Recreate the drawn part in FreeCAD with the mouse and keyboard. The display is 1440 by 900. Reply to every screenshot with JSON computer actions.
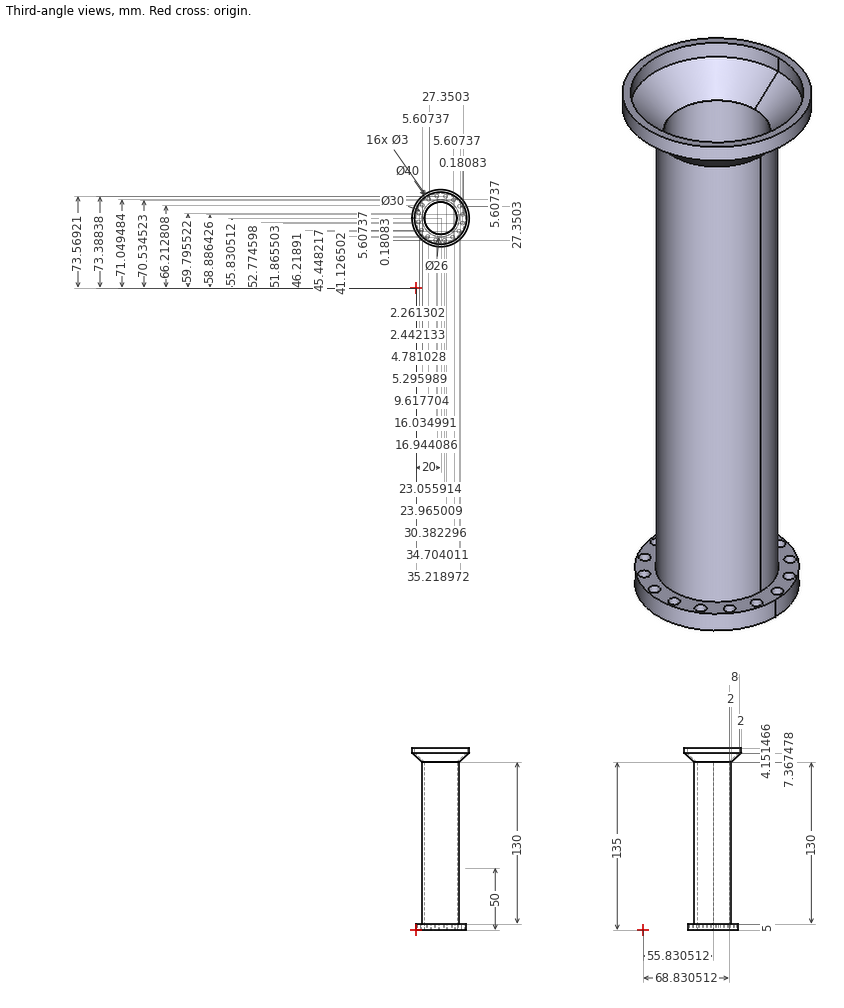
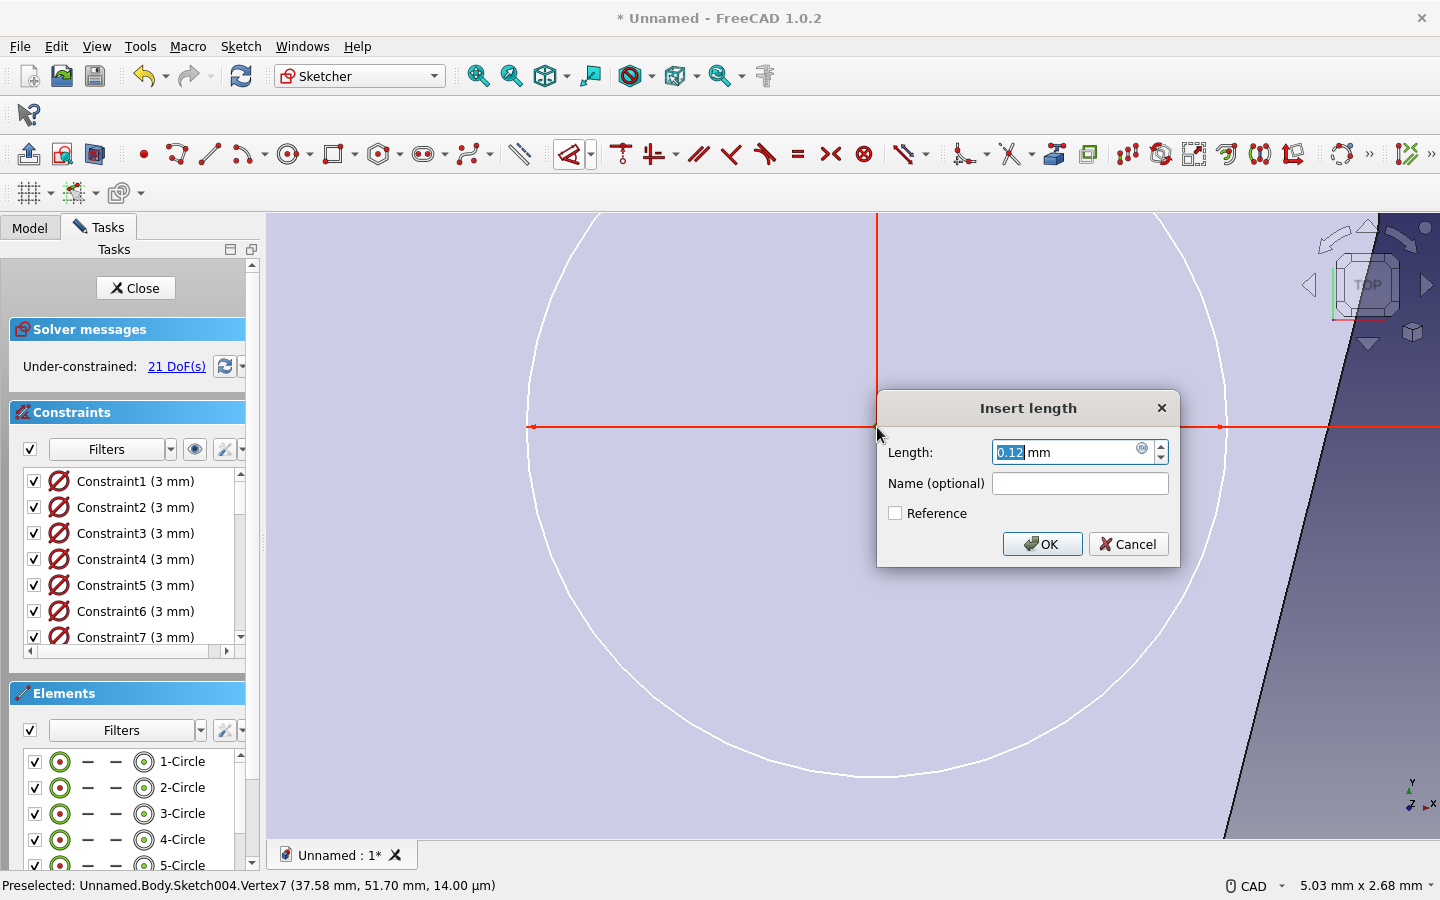
{"action": "type", "text": "0.18083"}
{"action": "key", "text": "Return"}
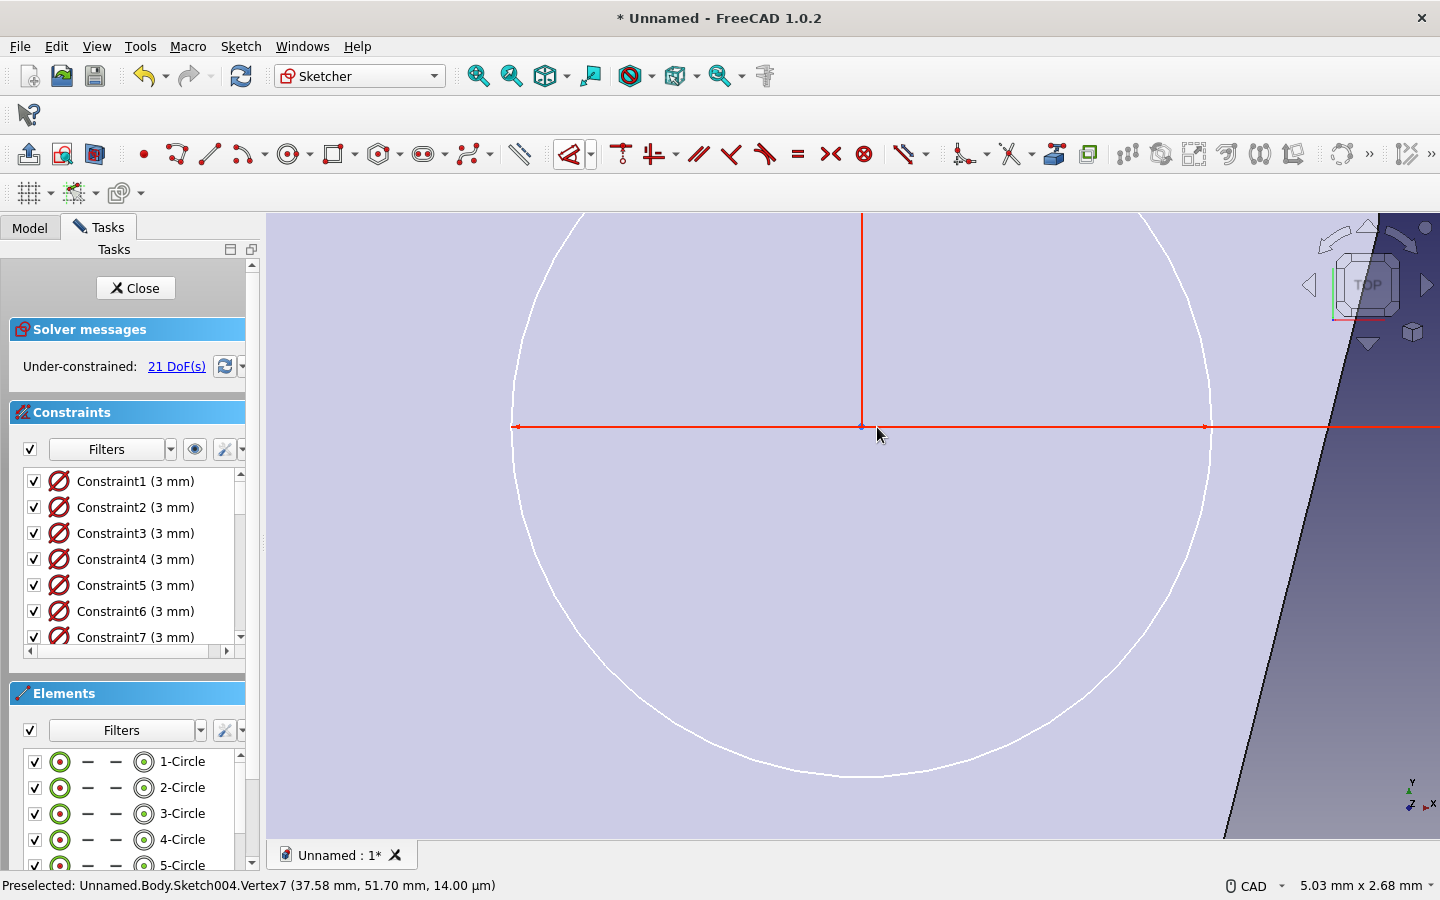
{"action": "scroll", "coordinate": [900, 436], "scroll_direction": "down", "scroll_amount": 18}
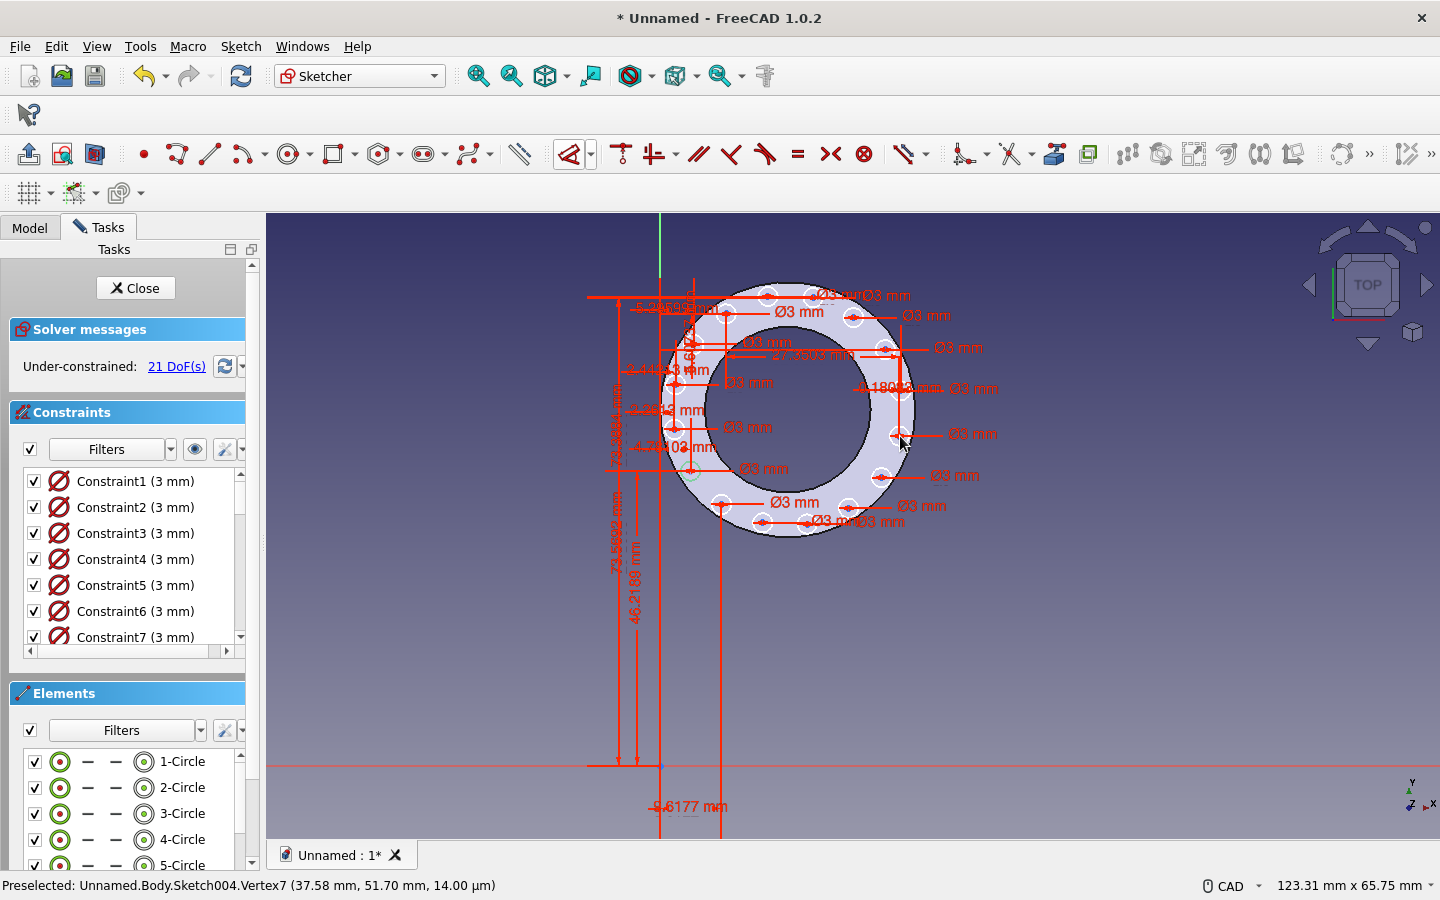
{"action": "left_click", "coordinate": [885, 350]}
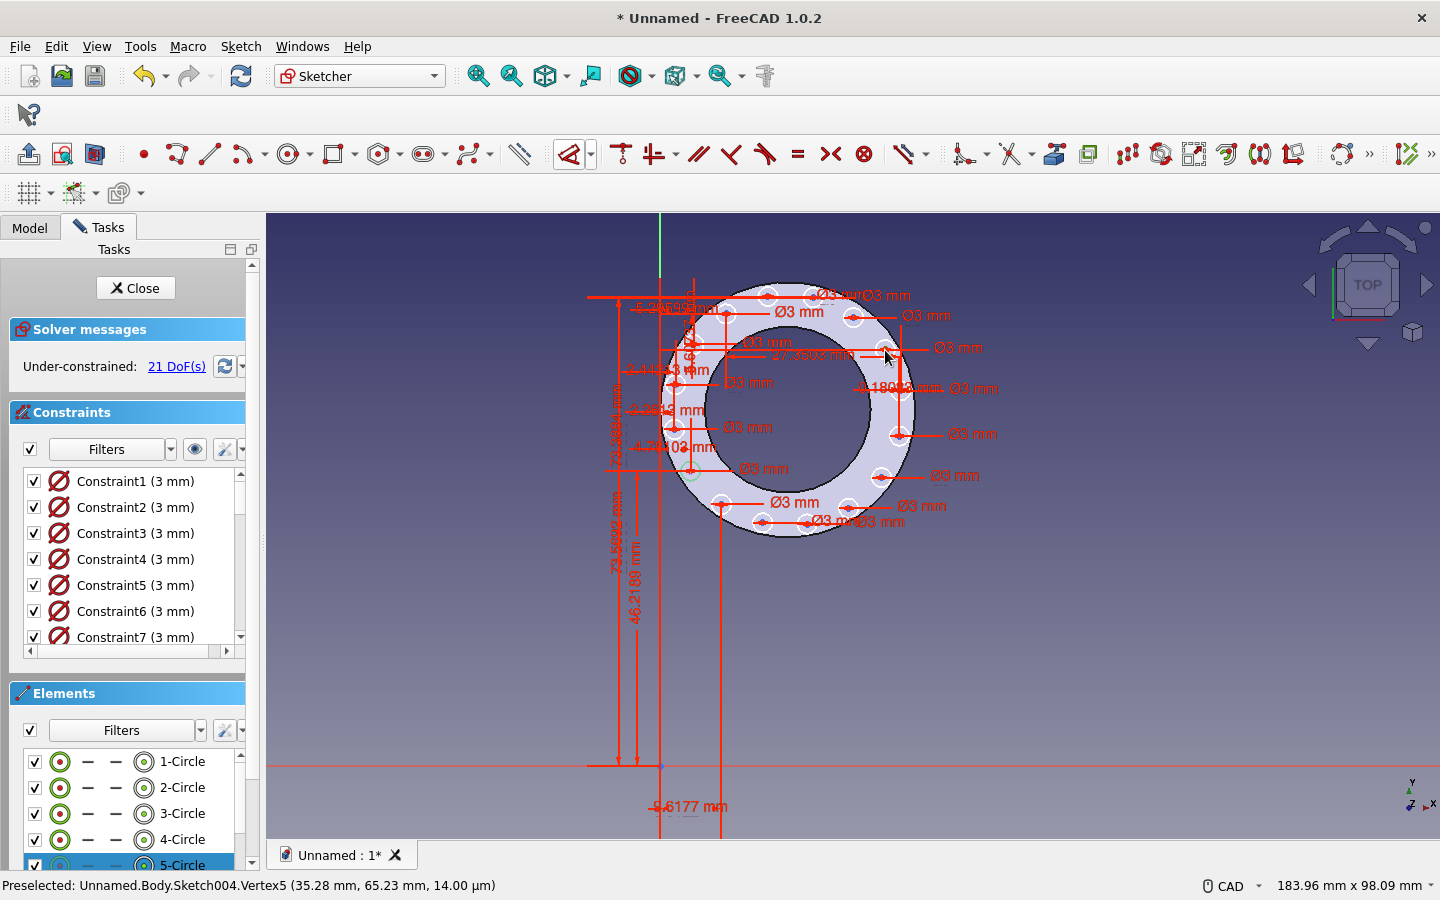
{"action": "left_click", "coordinate": [849, 508]}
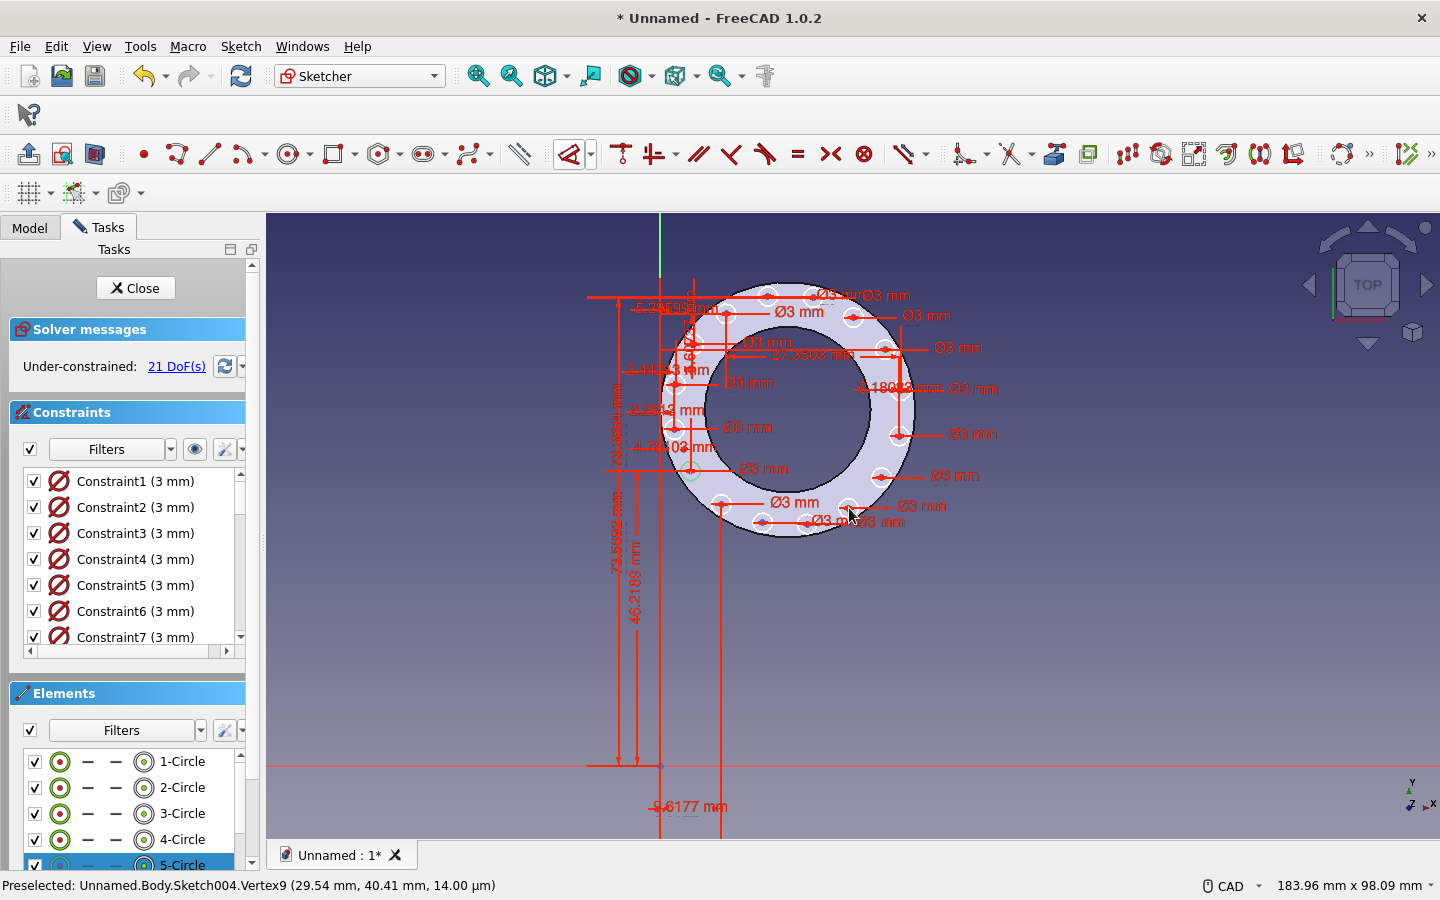
{"action": "key", "text": "l"}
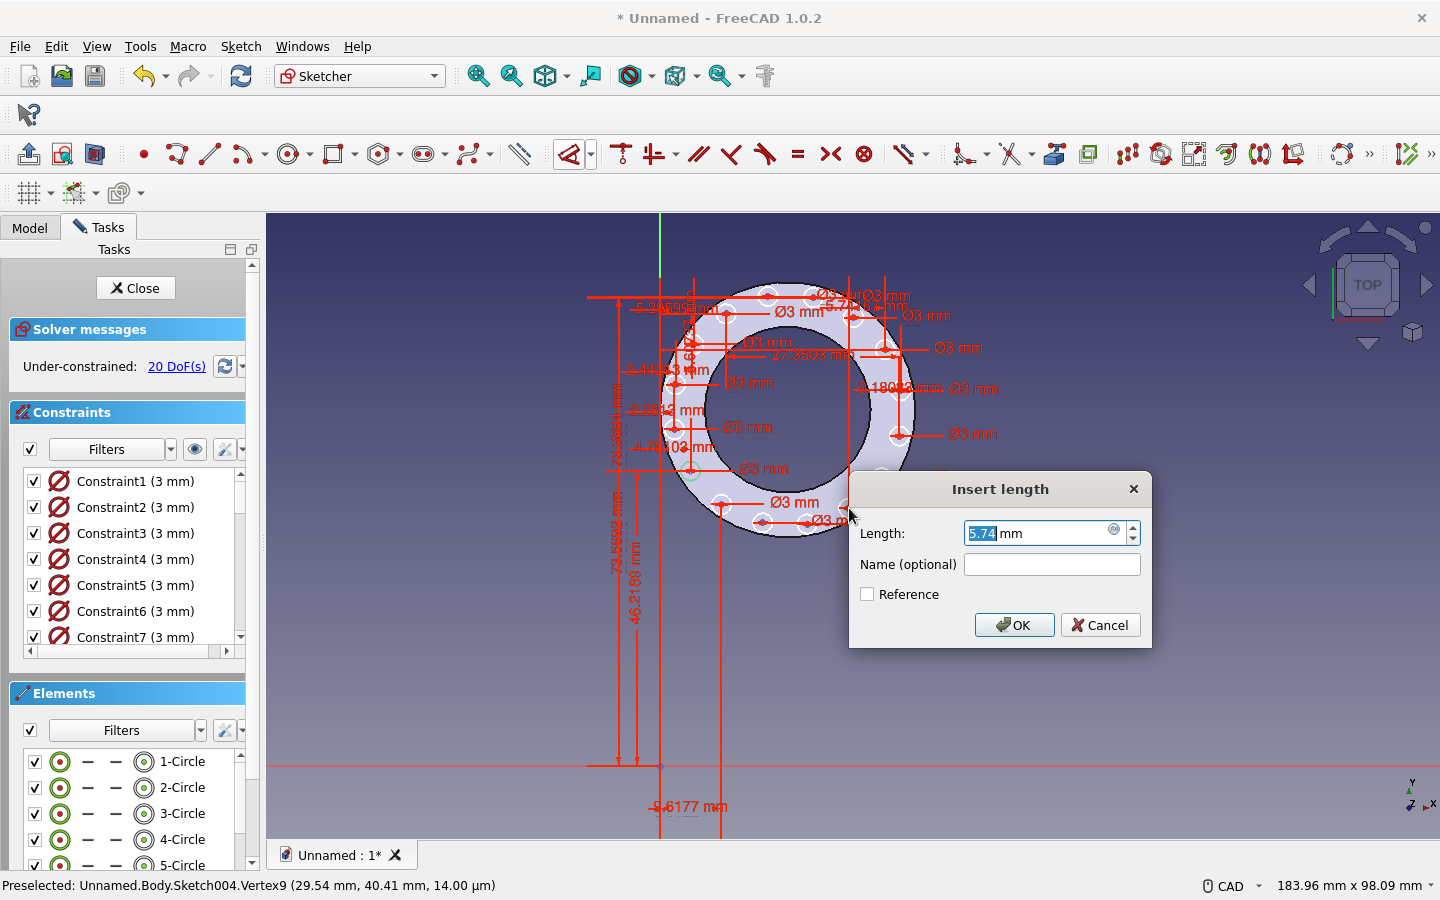
{"action": "type", "text": "5.60737"}
{"action": "key", "text": "Return"}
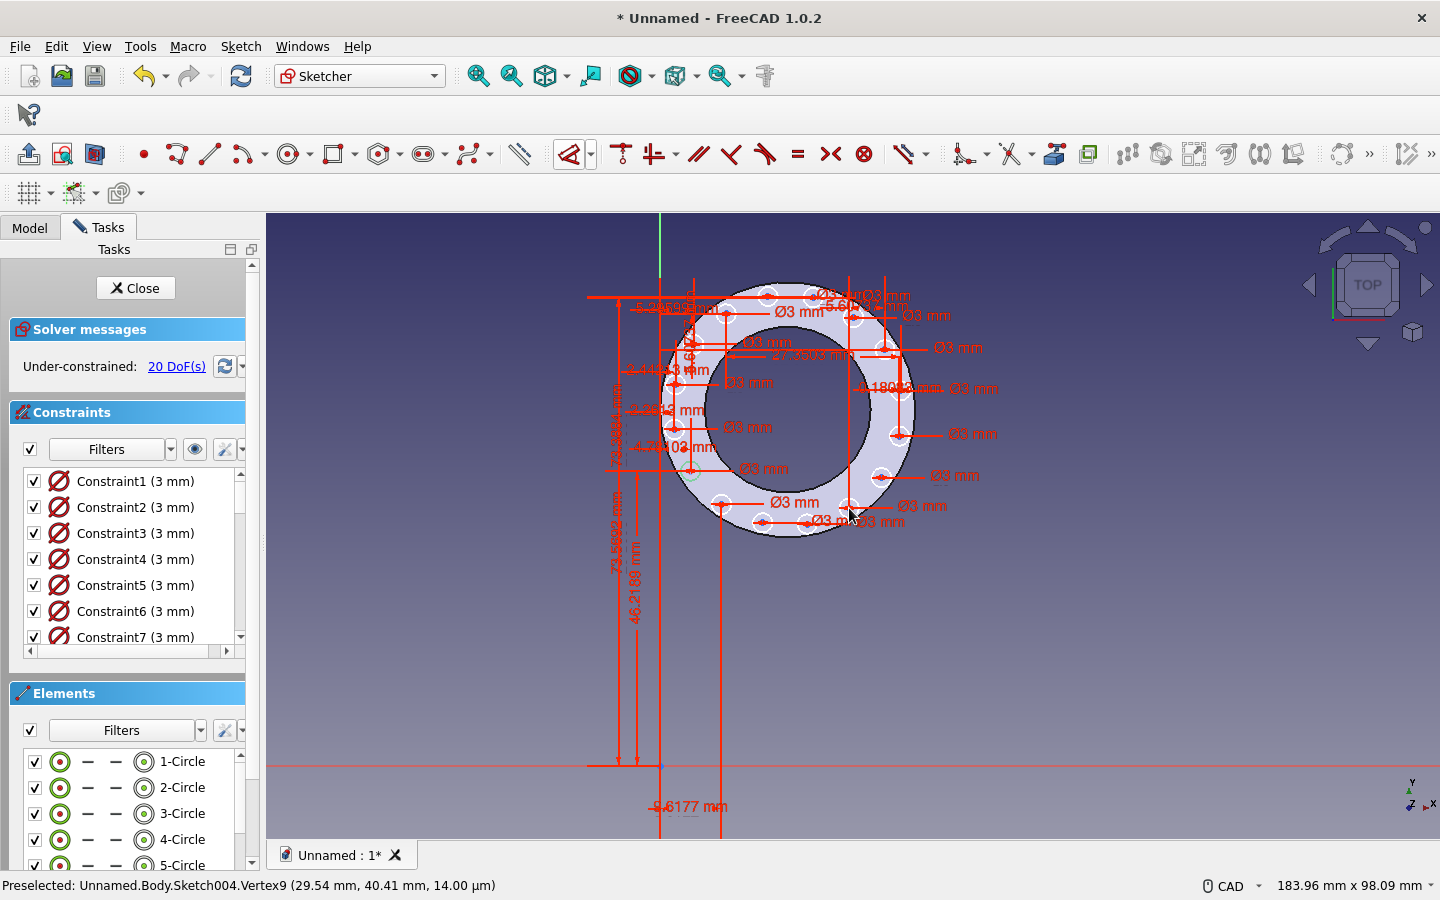
{"action": "left_click", "coordinate": [885, 350]}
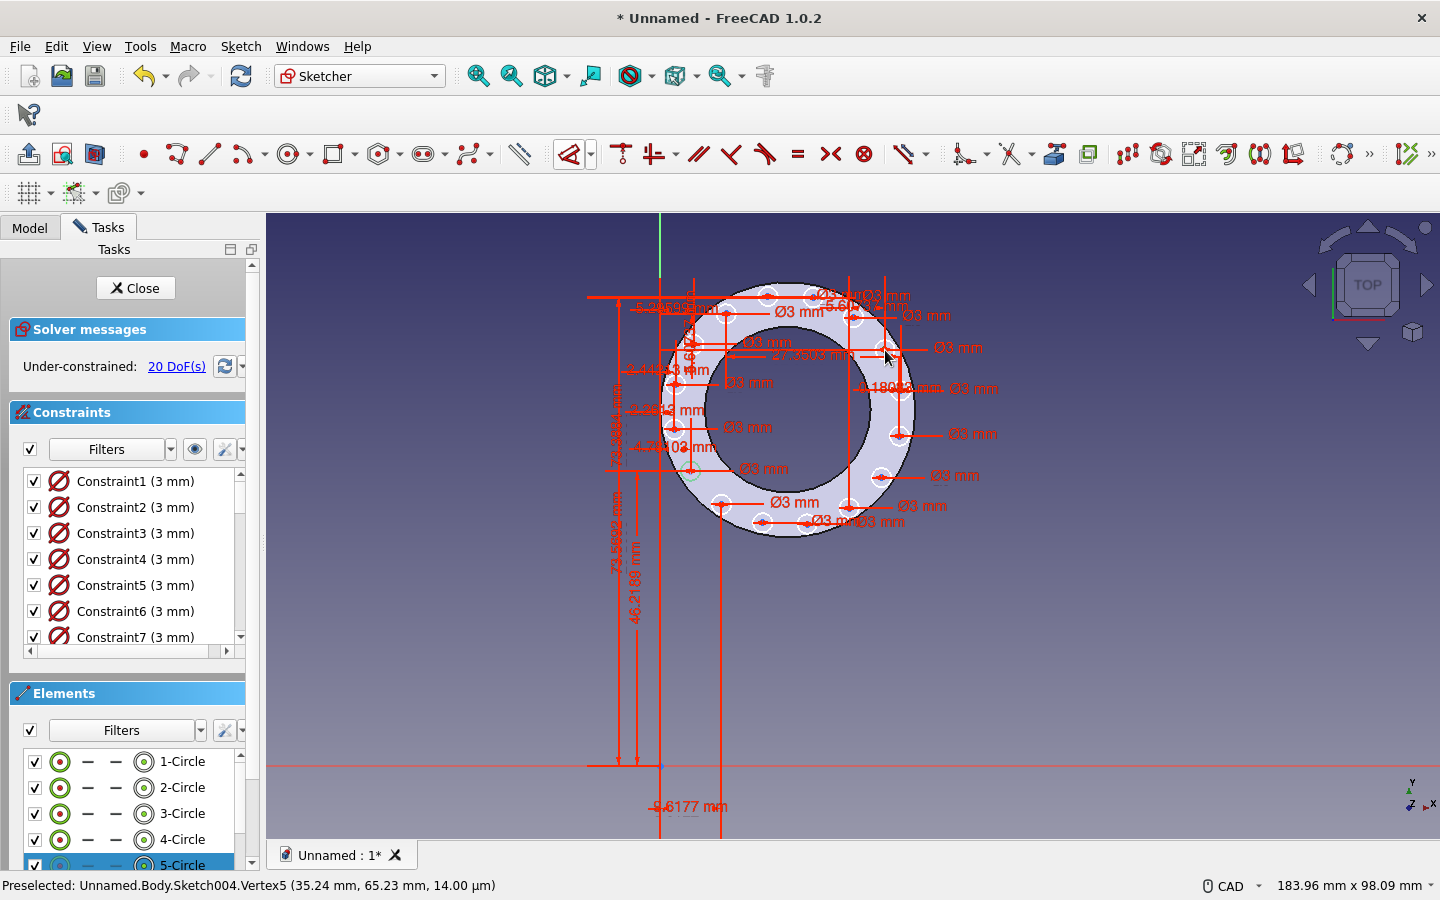
{"action": "left_click", "coordinate": [807, 524]}